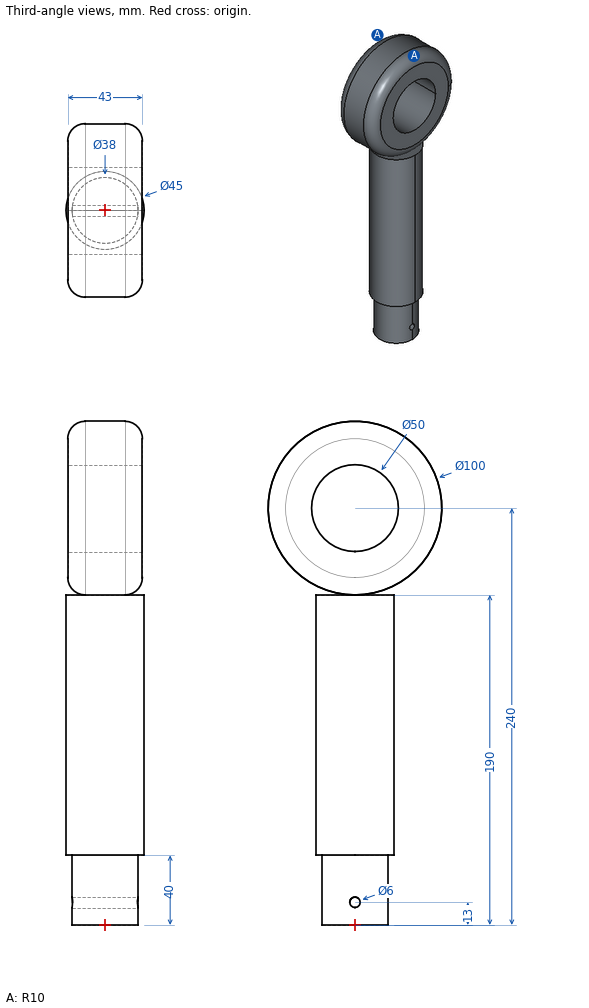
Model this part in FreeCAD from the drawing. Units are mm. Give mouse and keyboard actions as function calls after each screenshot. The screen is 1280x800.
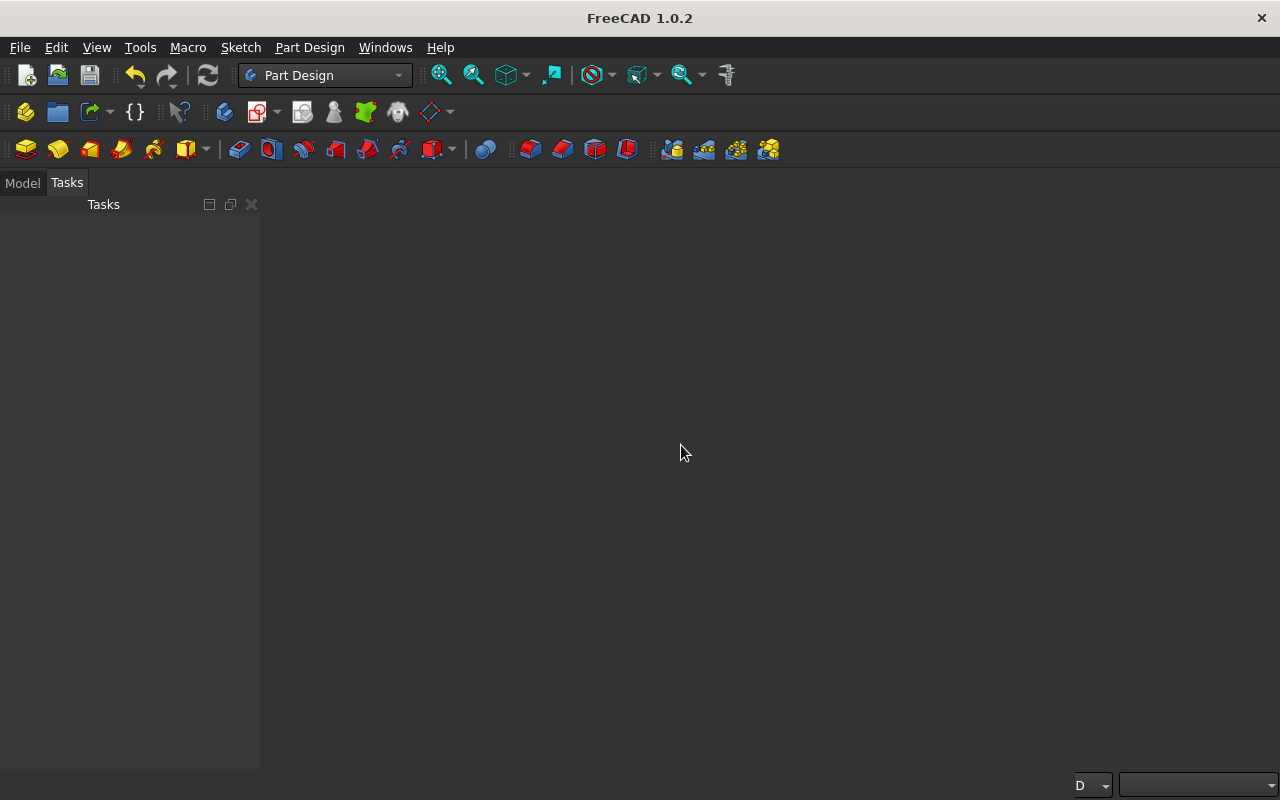
key(ctrl+n)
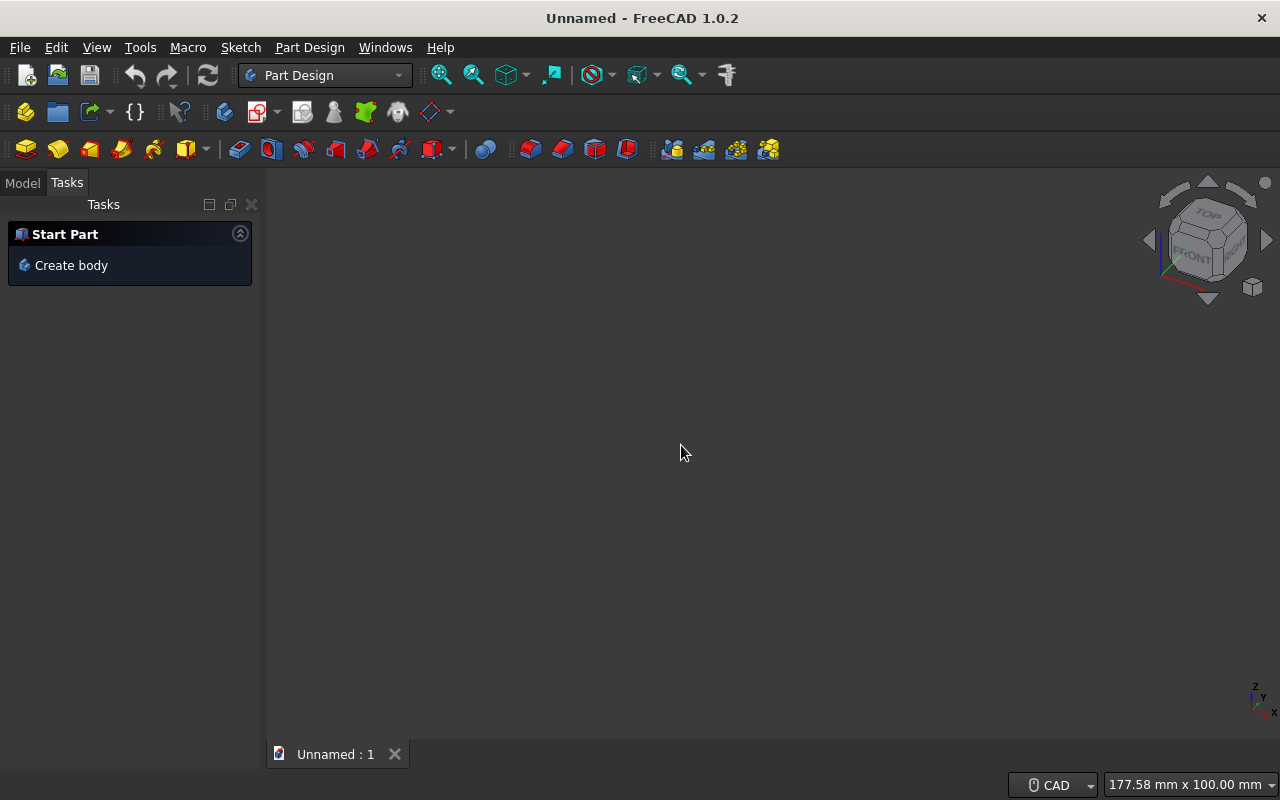
click(258, 112)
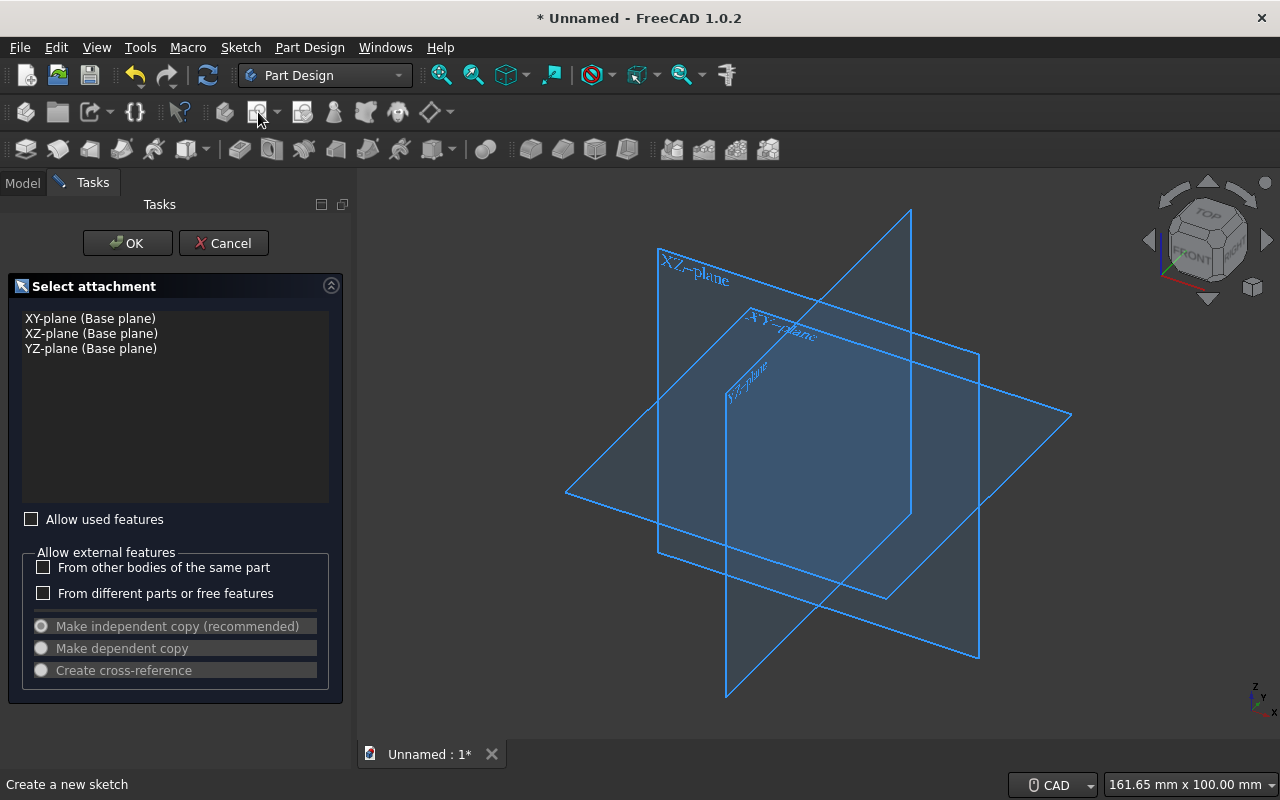
click(82, 318)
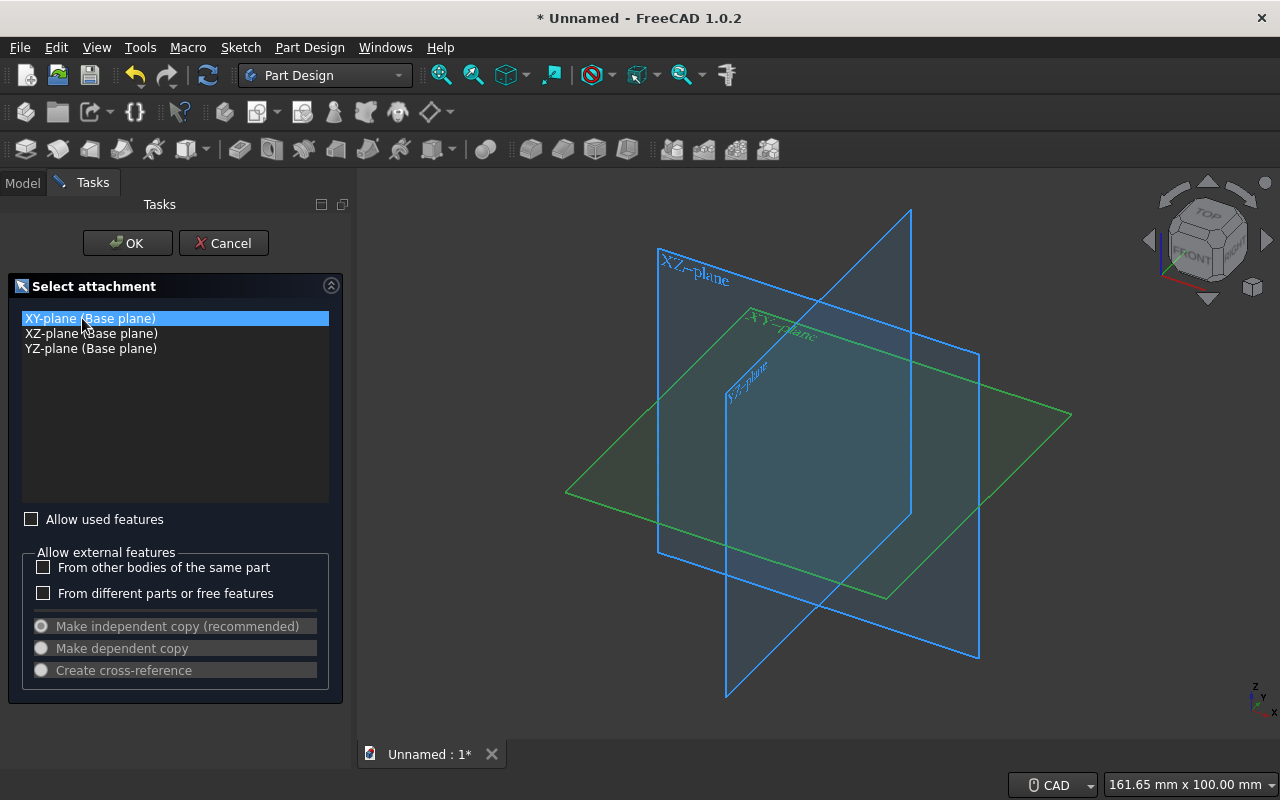
click(128, 243)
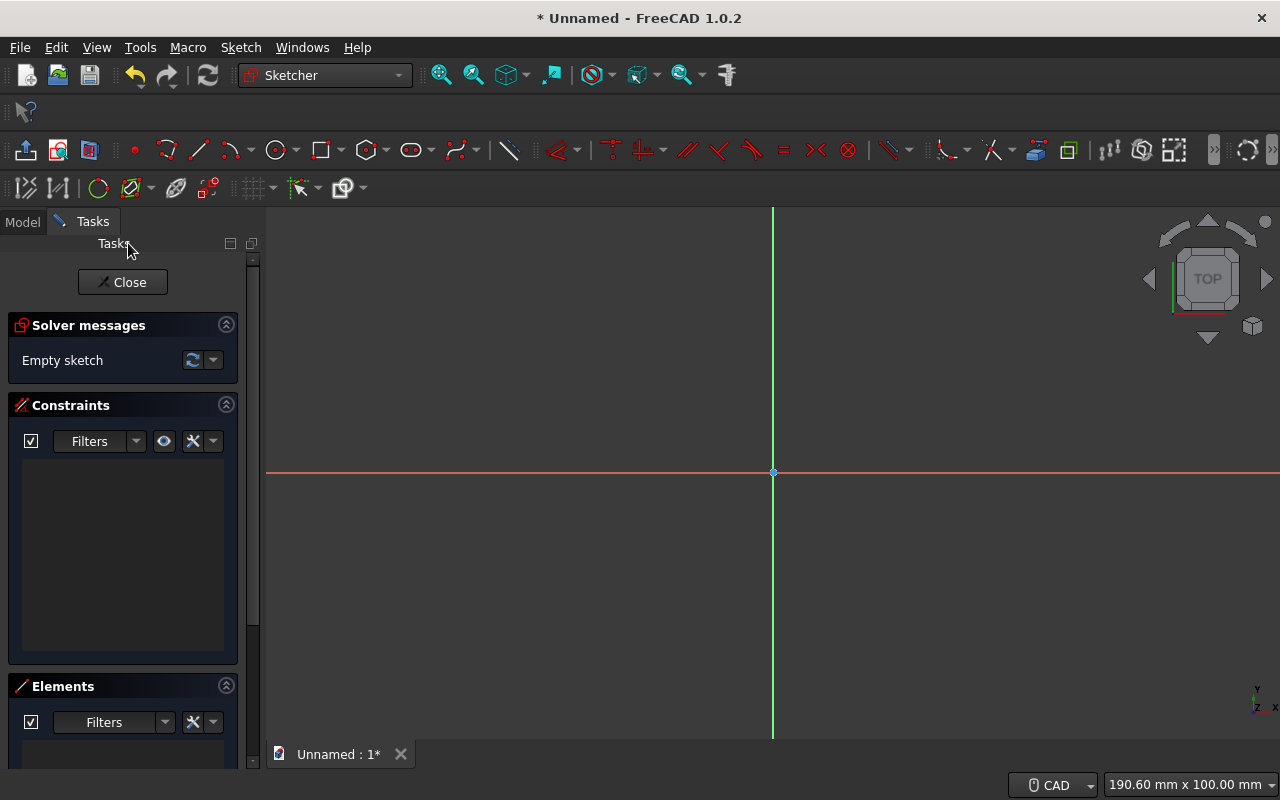
scroll(912, 473, up, 2)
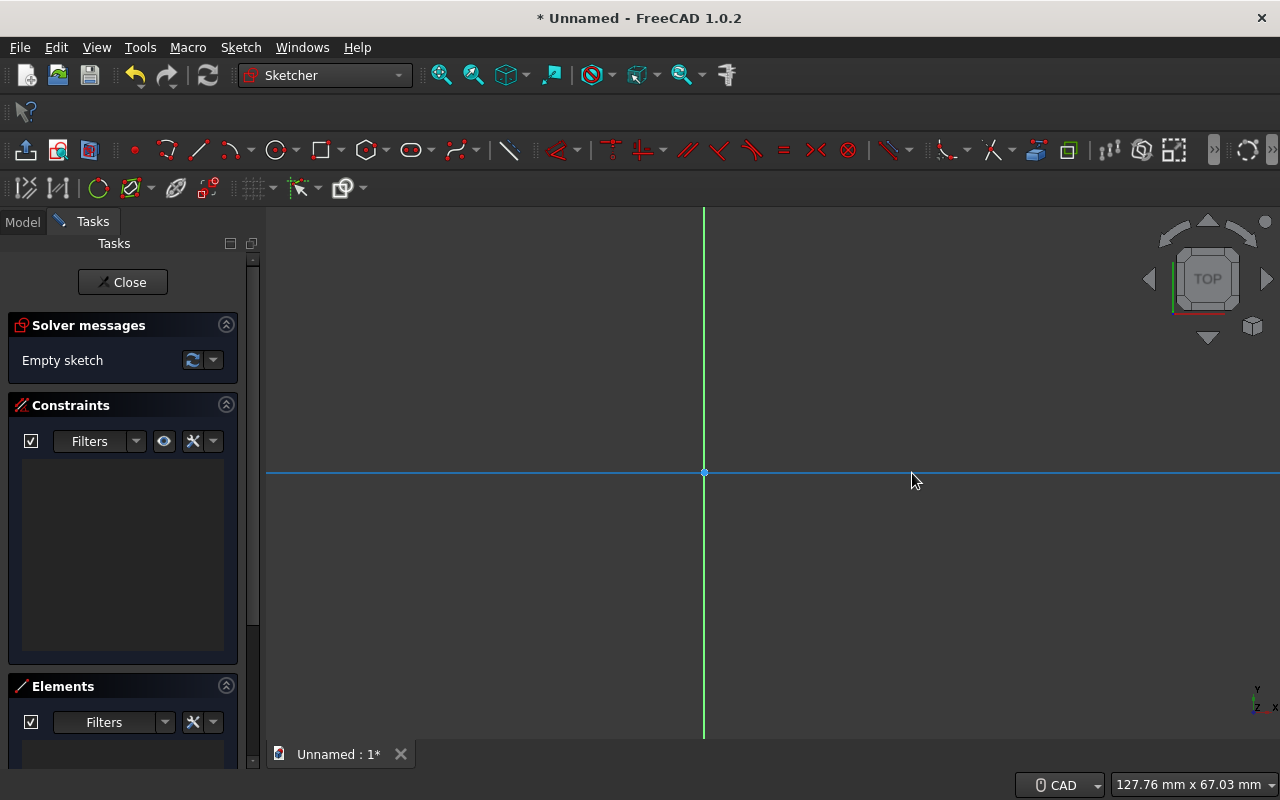
key(g)
key(c)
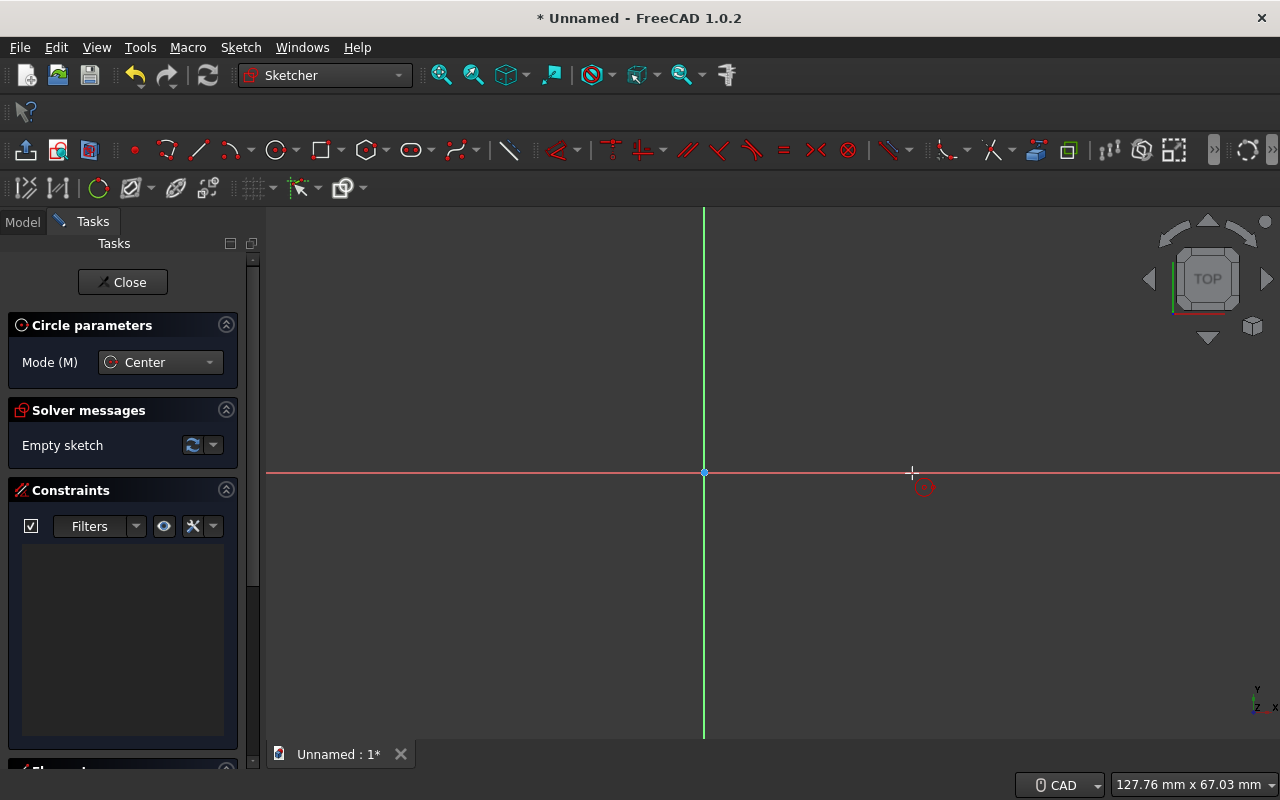
click(704, 473)
move(831, 346)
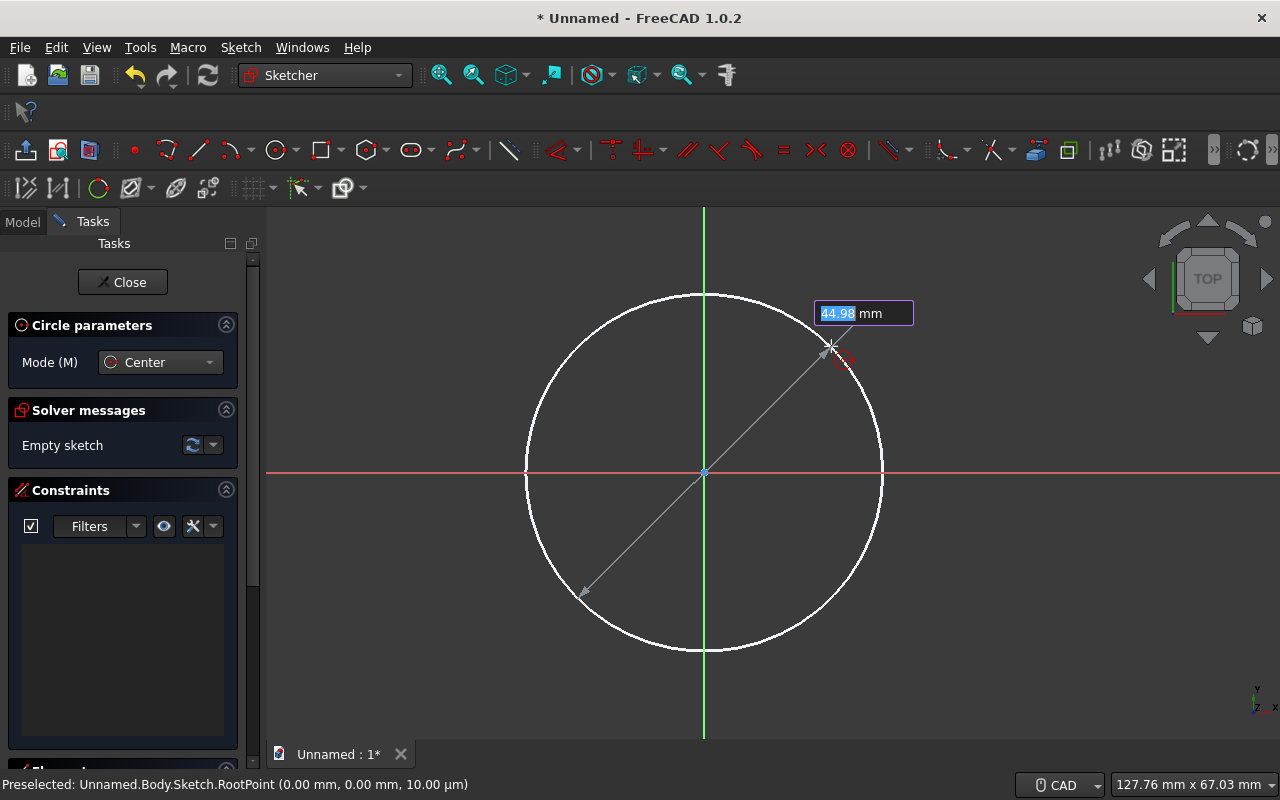
text(45)
key(Return)
key(Escape)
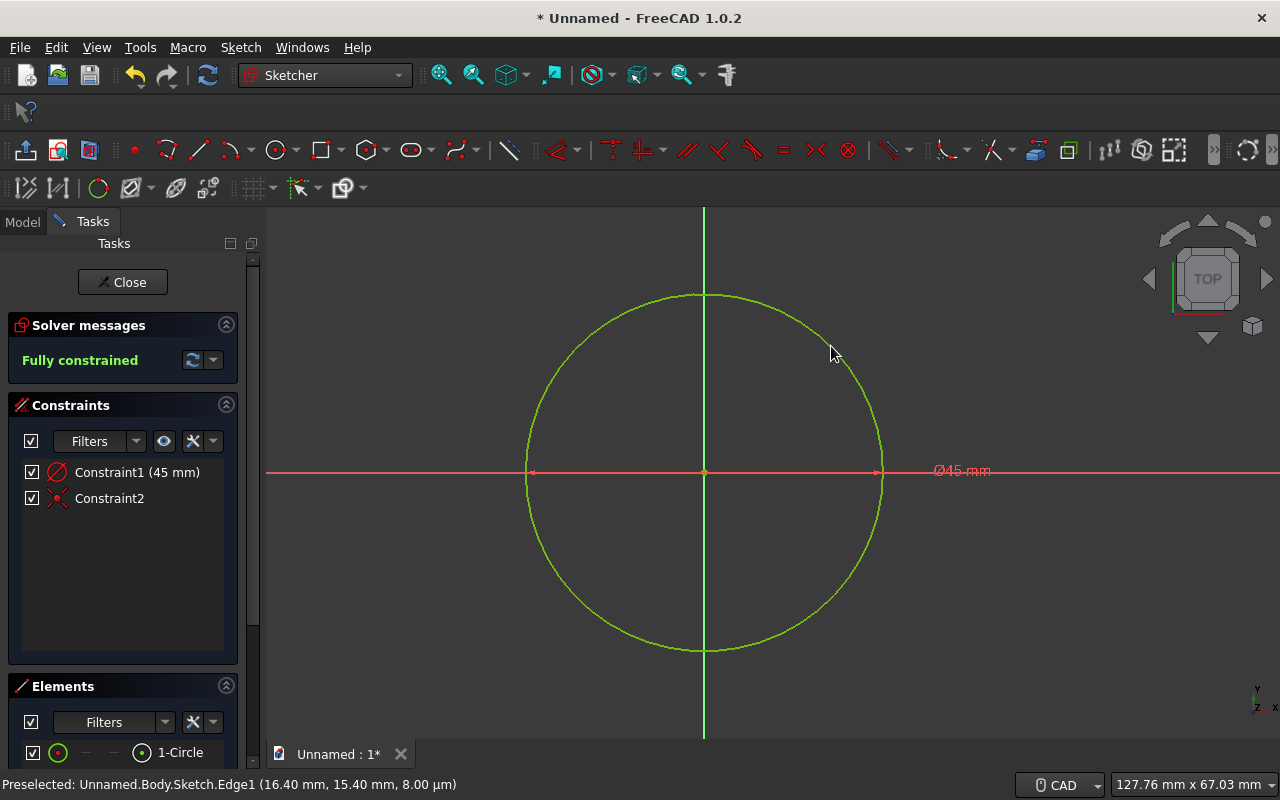
click(123, 282)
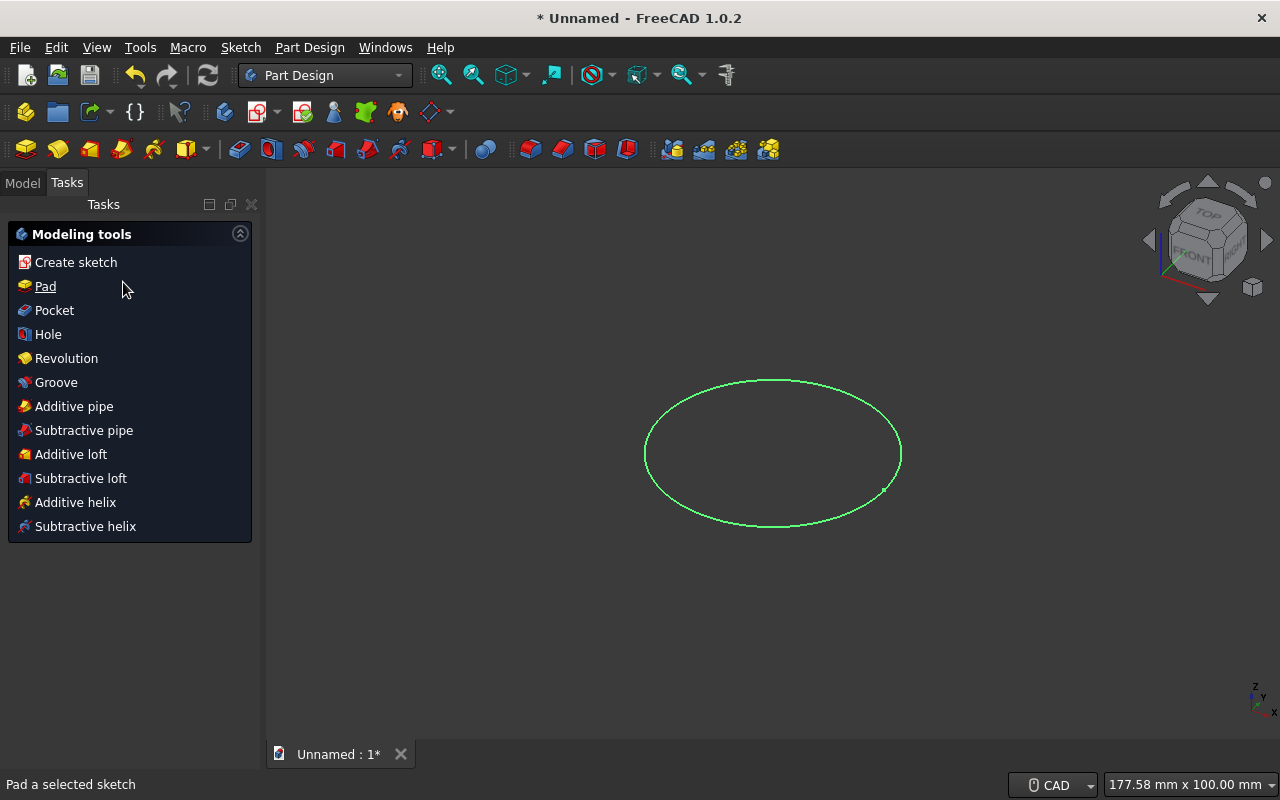
click(26, 150)